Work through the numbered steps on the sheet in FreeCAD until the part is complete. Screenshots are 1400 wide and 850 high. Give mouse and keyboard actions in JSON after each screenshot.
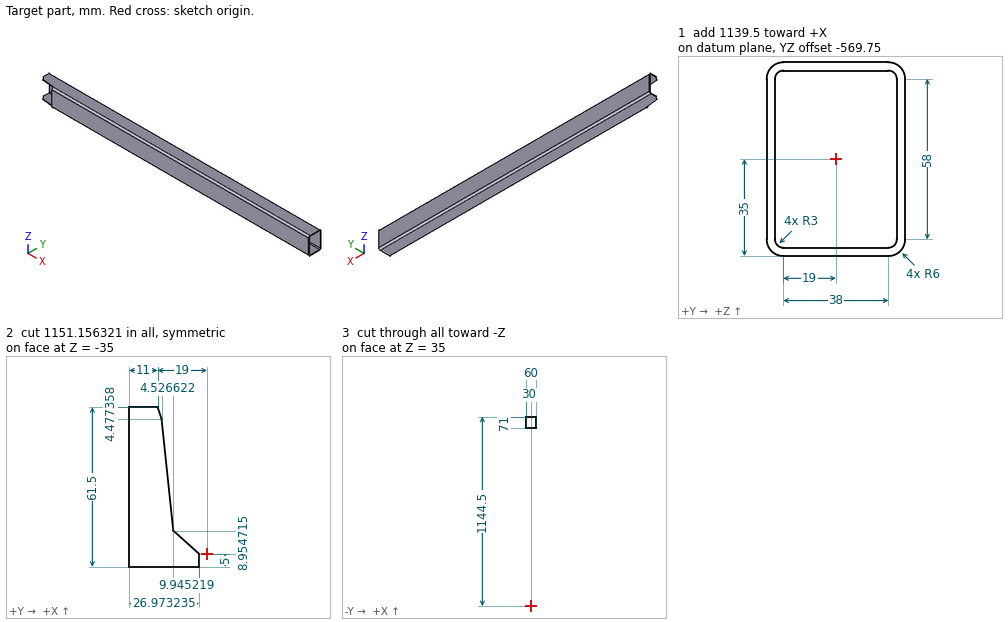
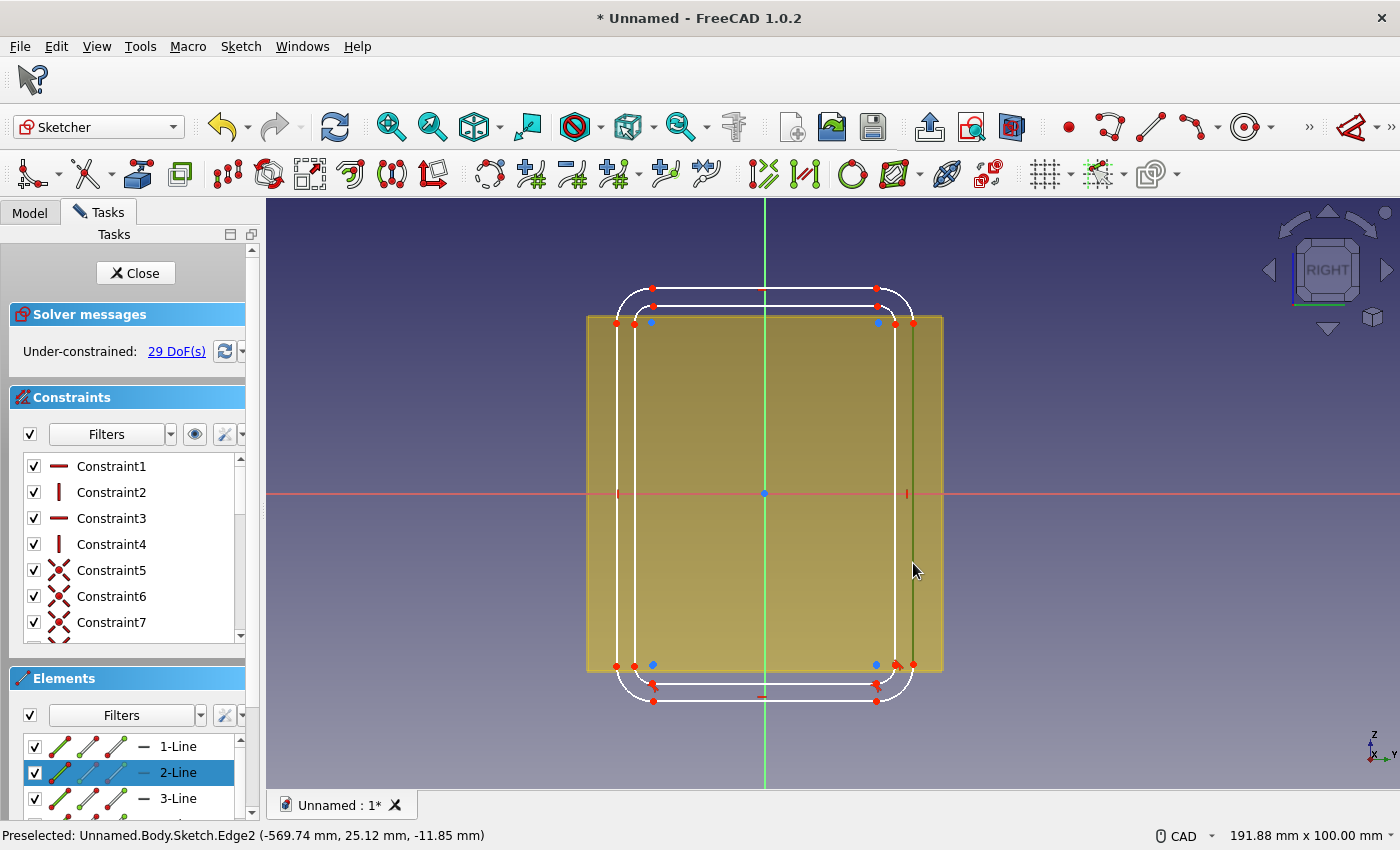
{"action": "left_click", "coordinate": [909, 307]}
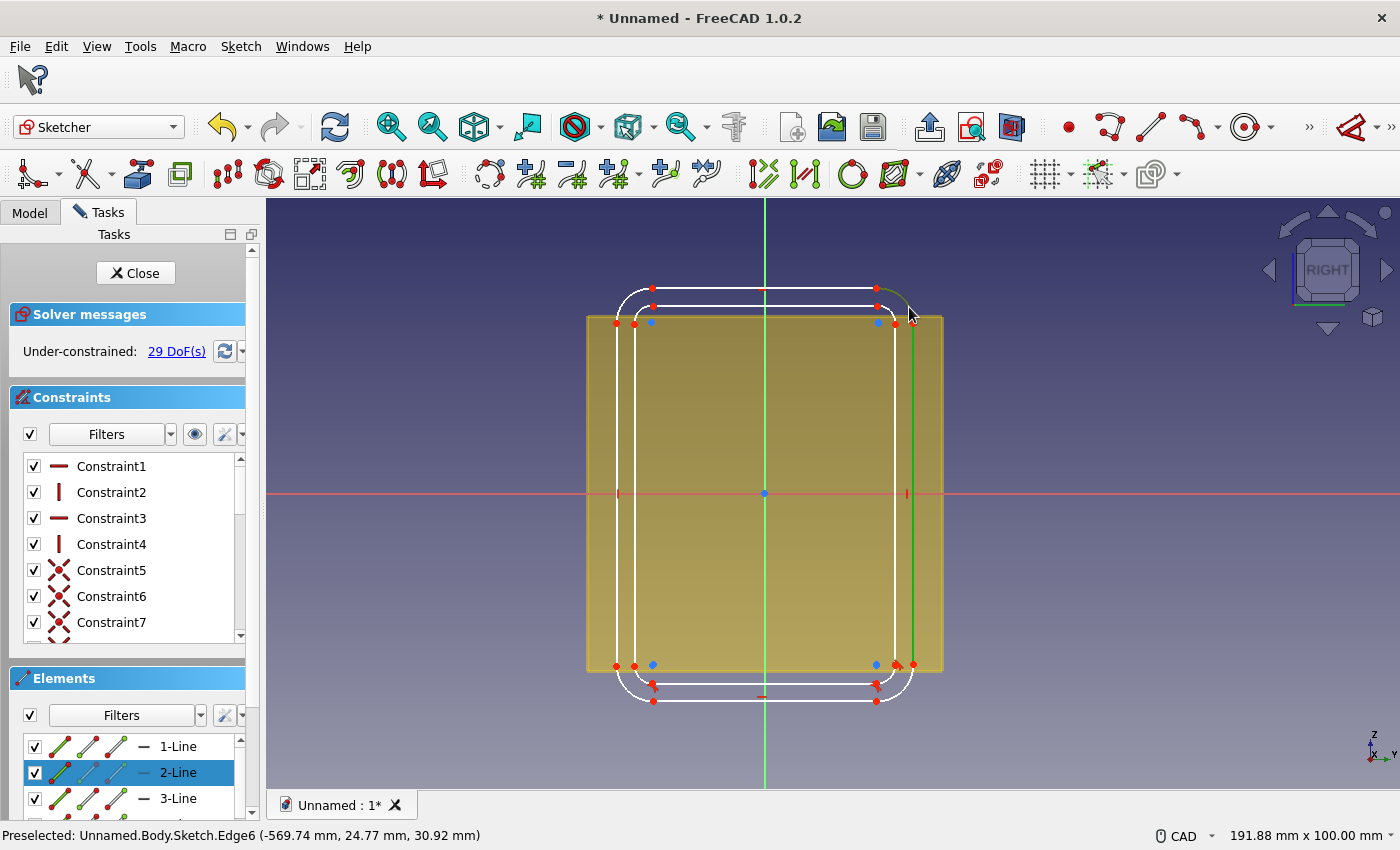
{"action": "key", "text": "t"}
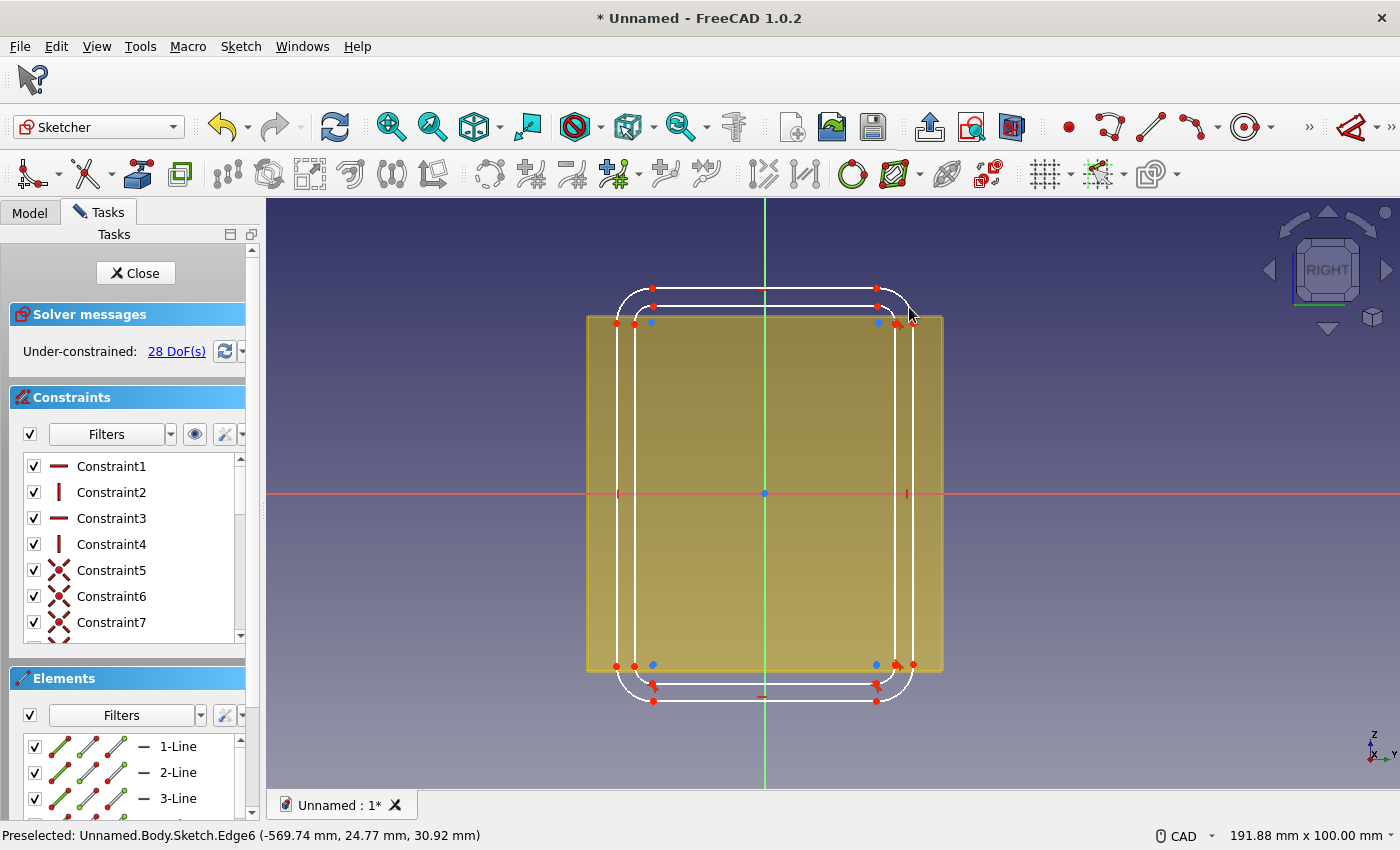
{"action": "left_click", "coordinate": [810, 288]}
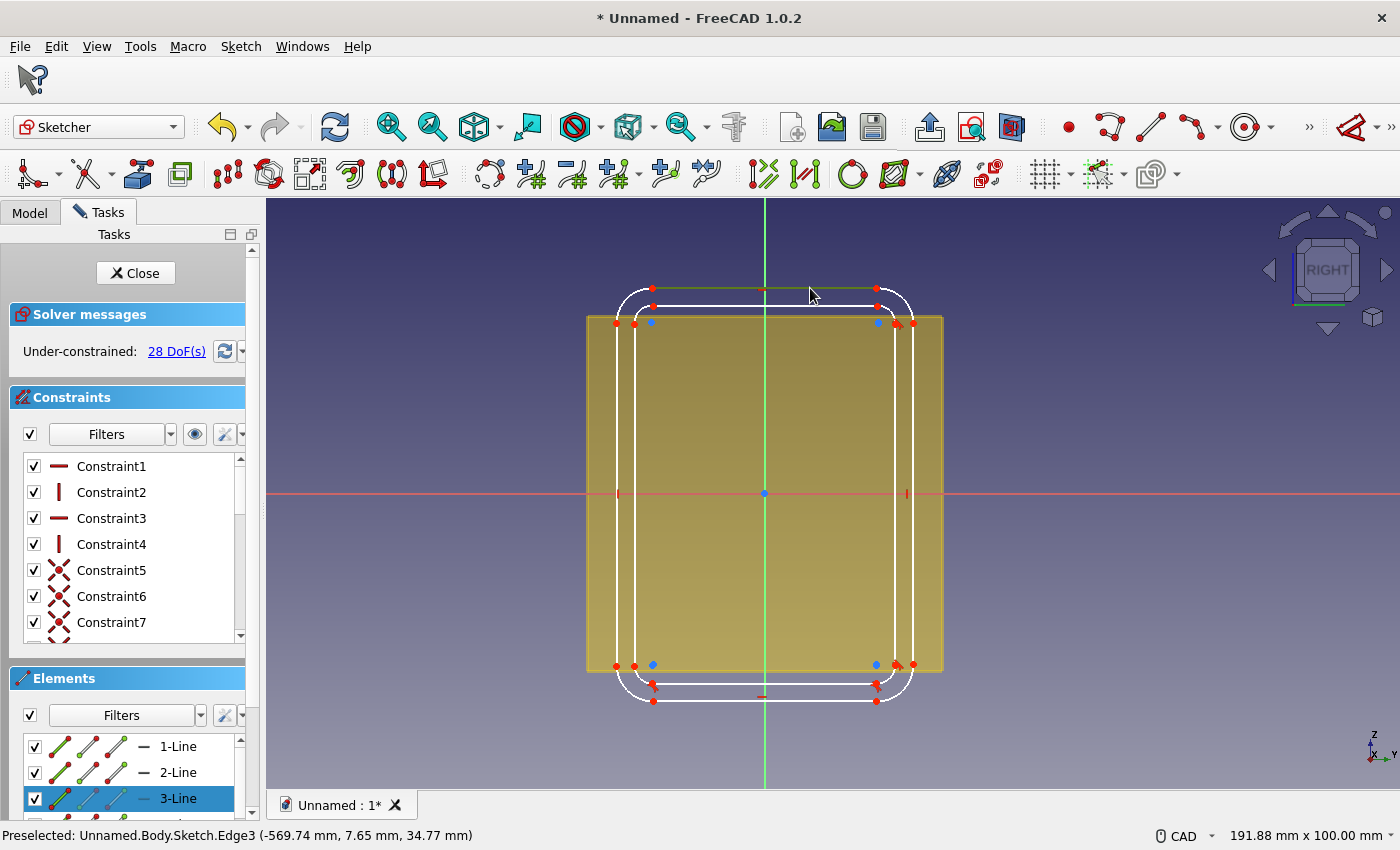
{"action": "left_click", "coordinate": [909, 307]}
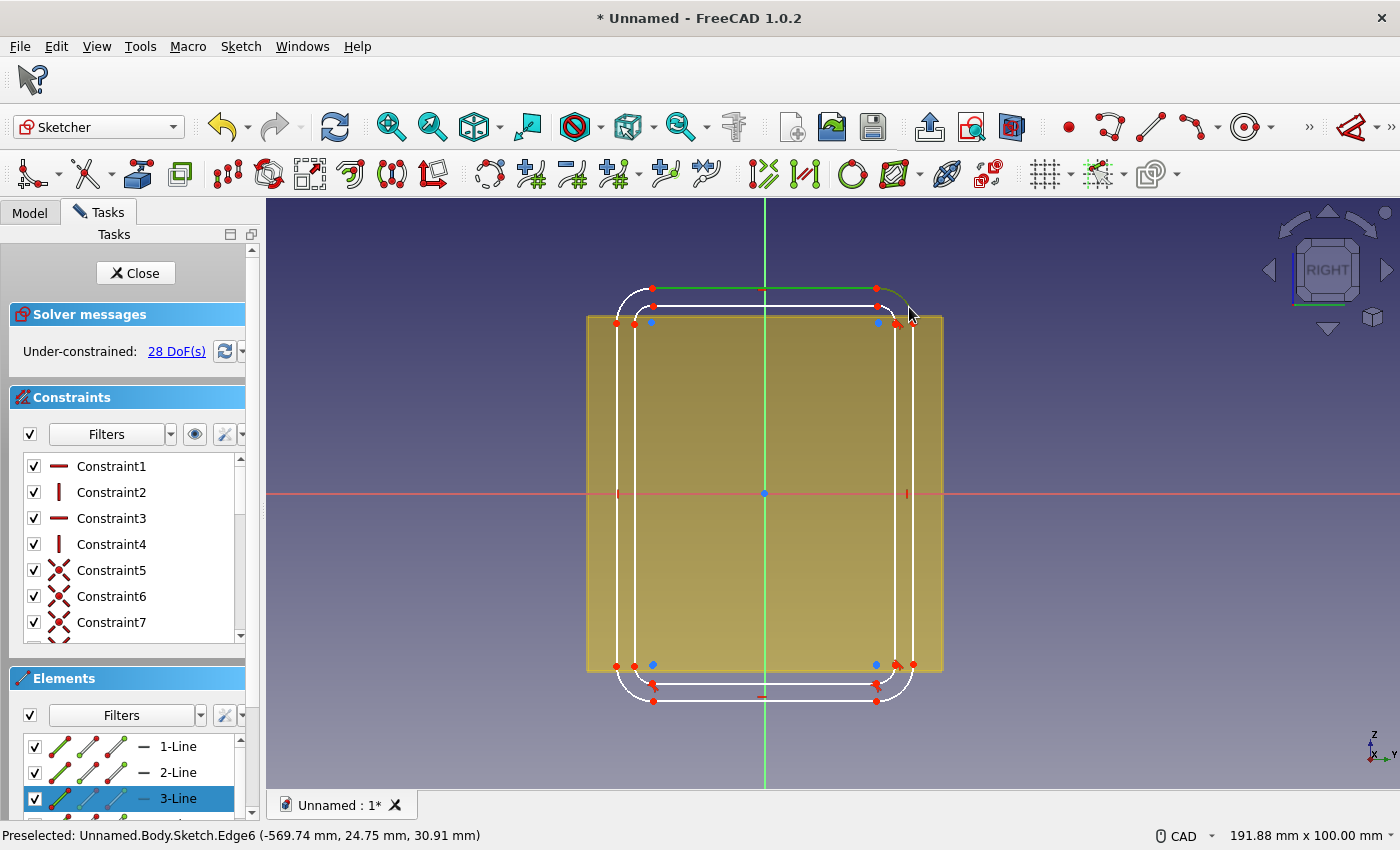
{"action": "key", "text": "t"}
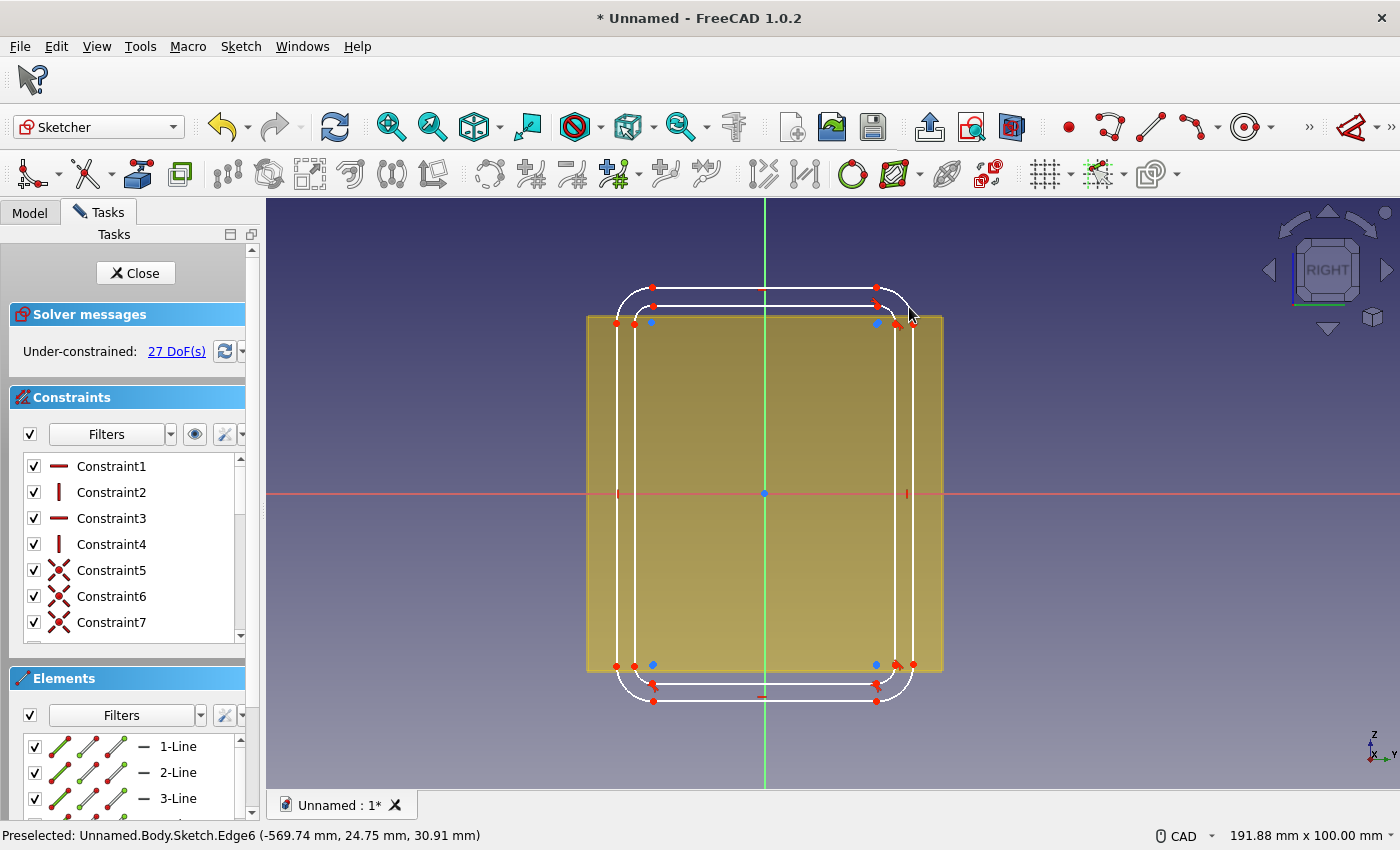
{"action": "left_click", "coordinate": [810, 288]}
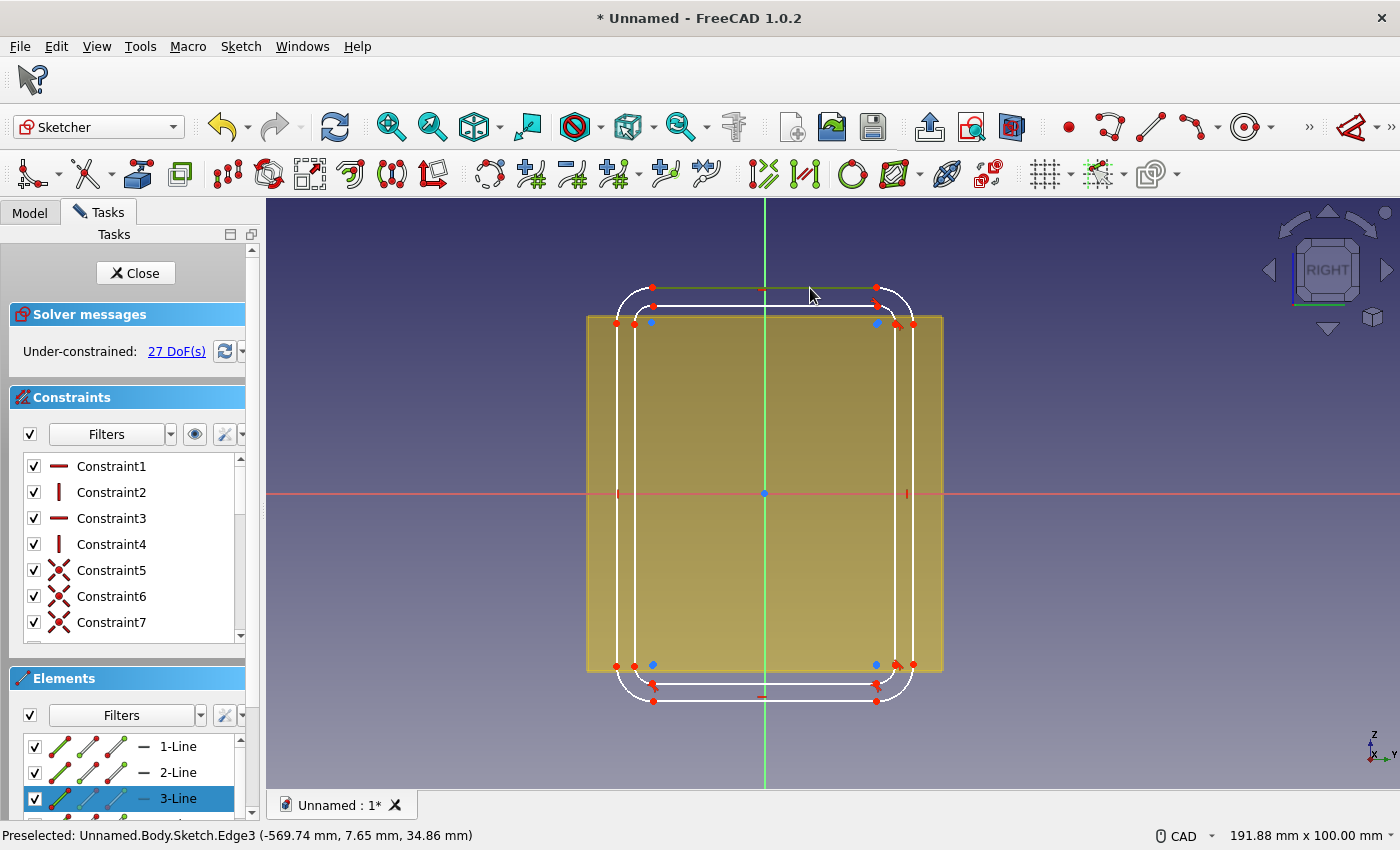
{"action": "left_click", "coordinate": [636, 291]}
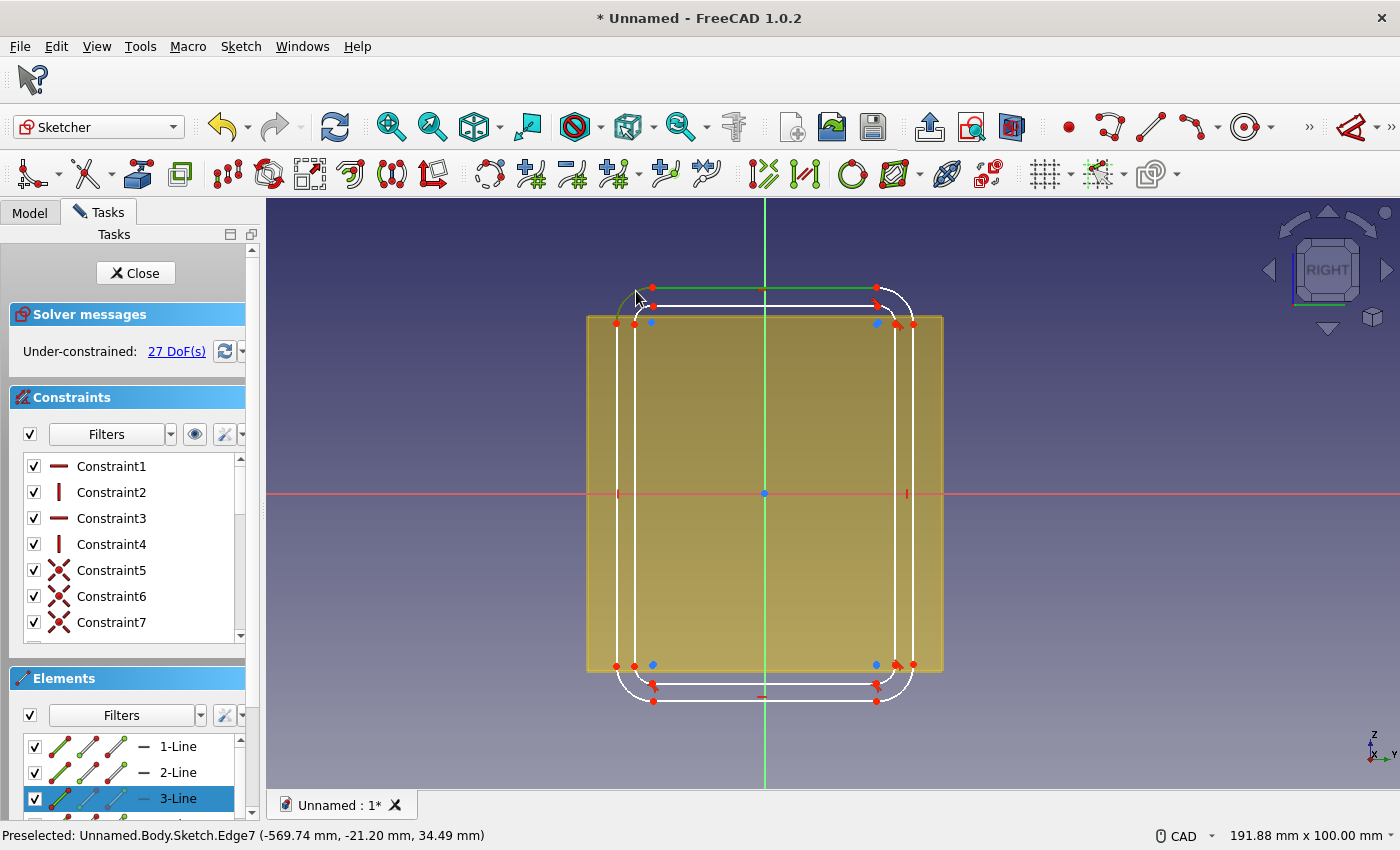
{"action": "key", "text": "t"}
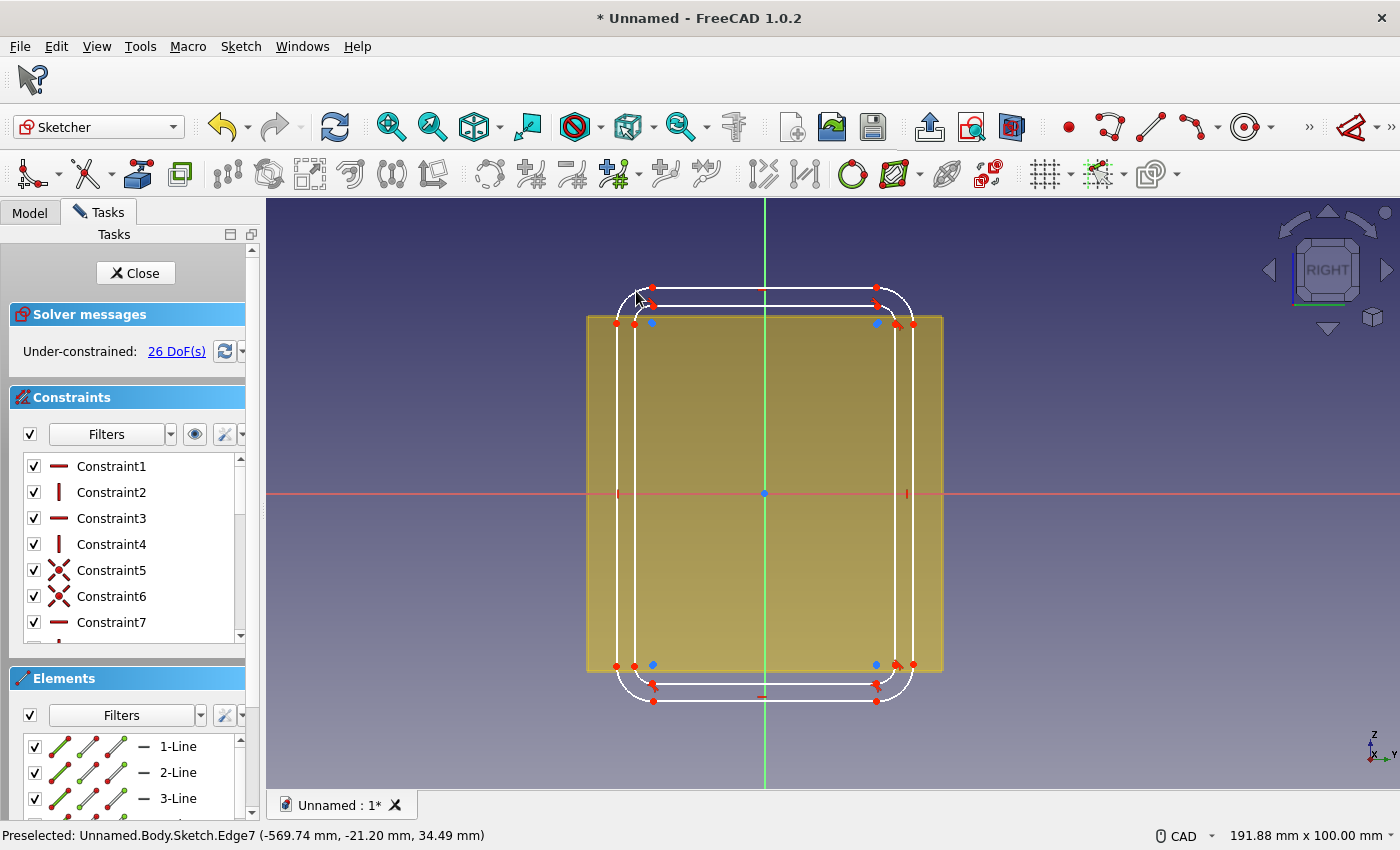
{"action": "left_click", "coordinate": [617, 426]}